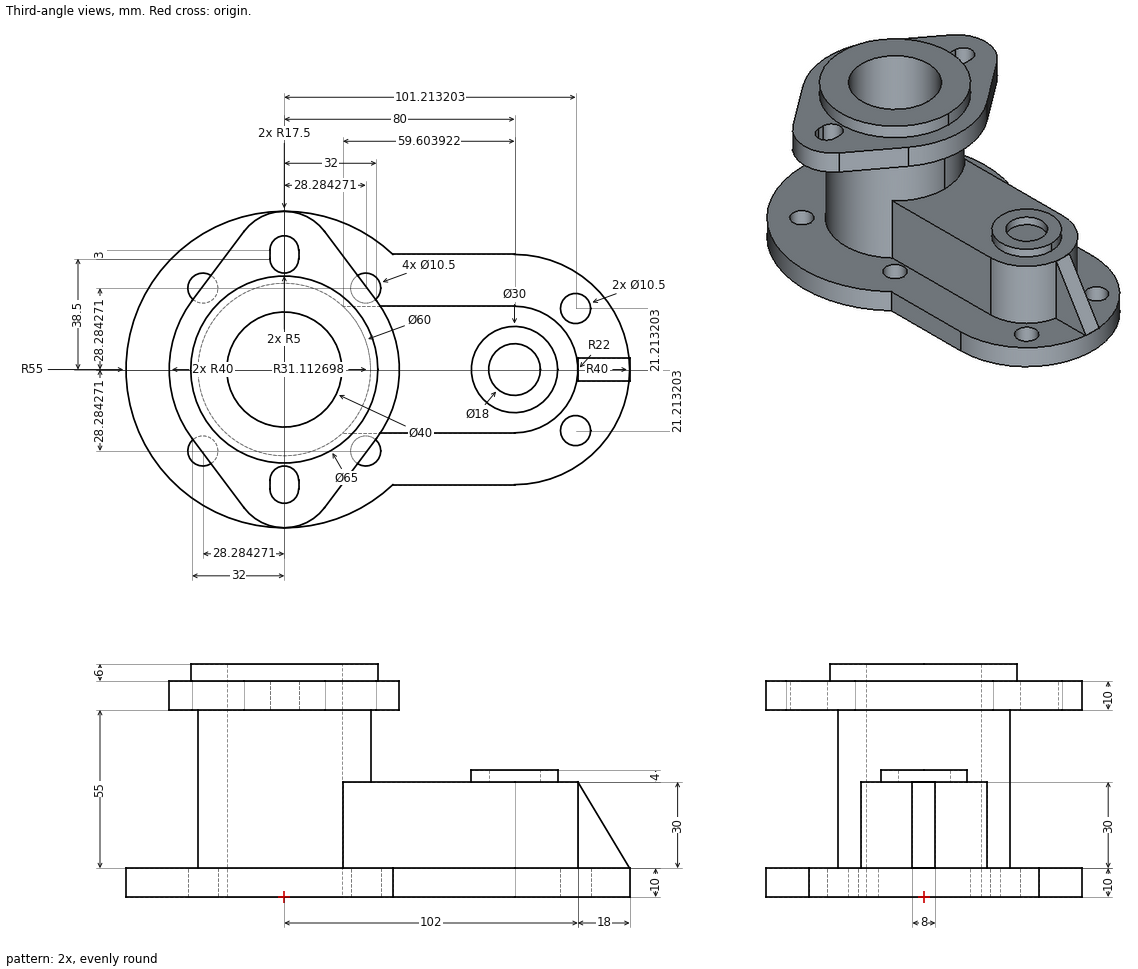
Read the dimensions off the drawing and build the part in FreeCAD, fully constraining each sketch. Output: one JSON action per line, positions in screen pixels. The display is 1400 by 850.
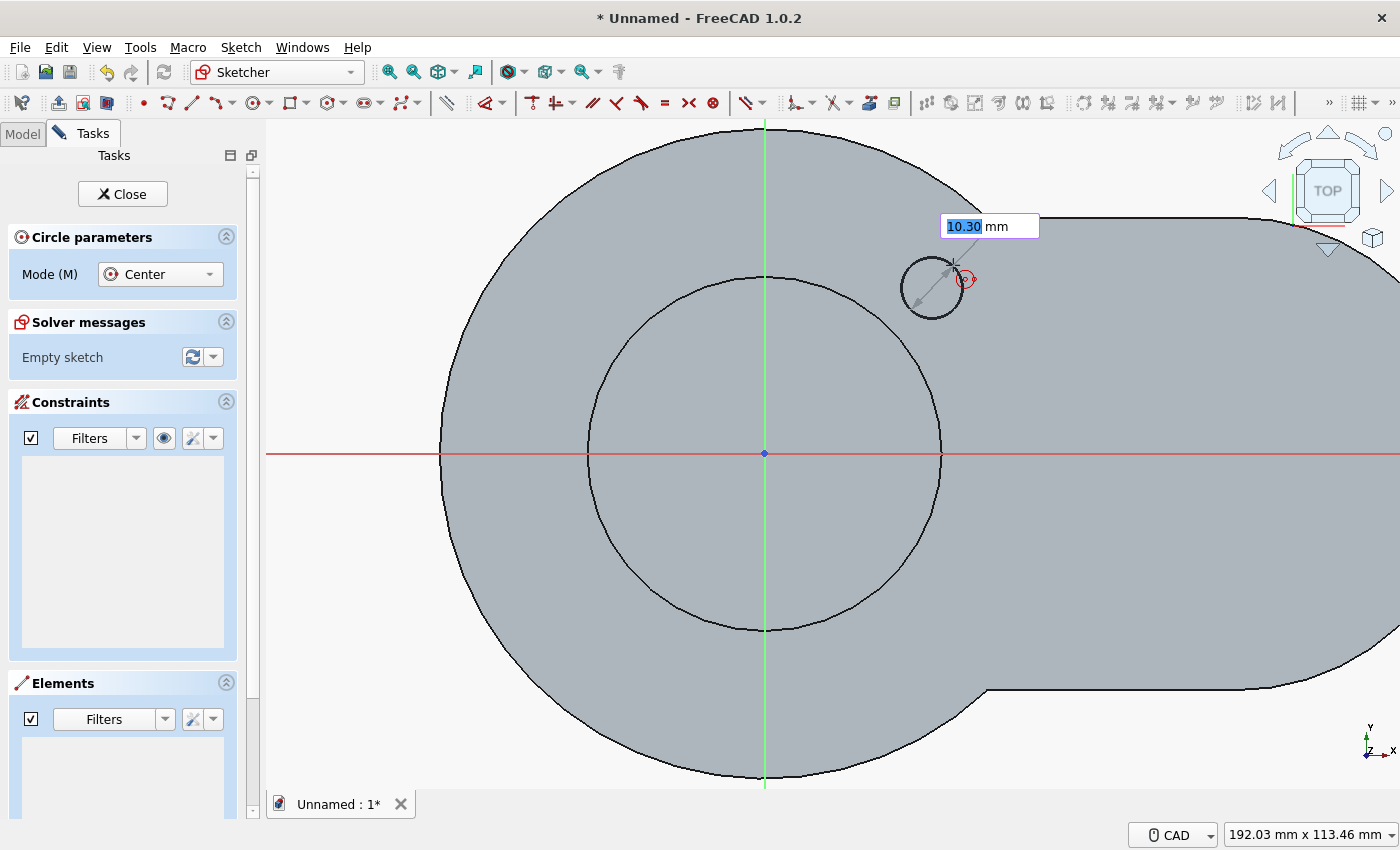
{"action": "type", "text": "10.5"}
{"action": "key", "text": "Return"}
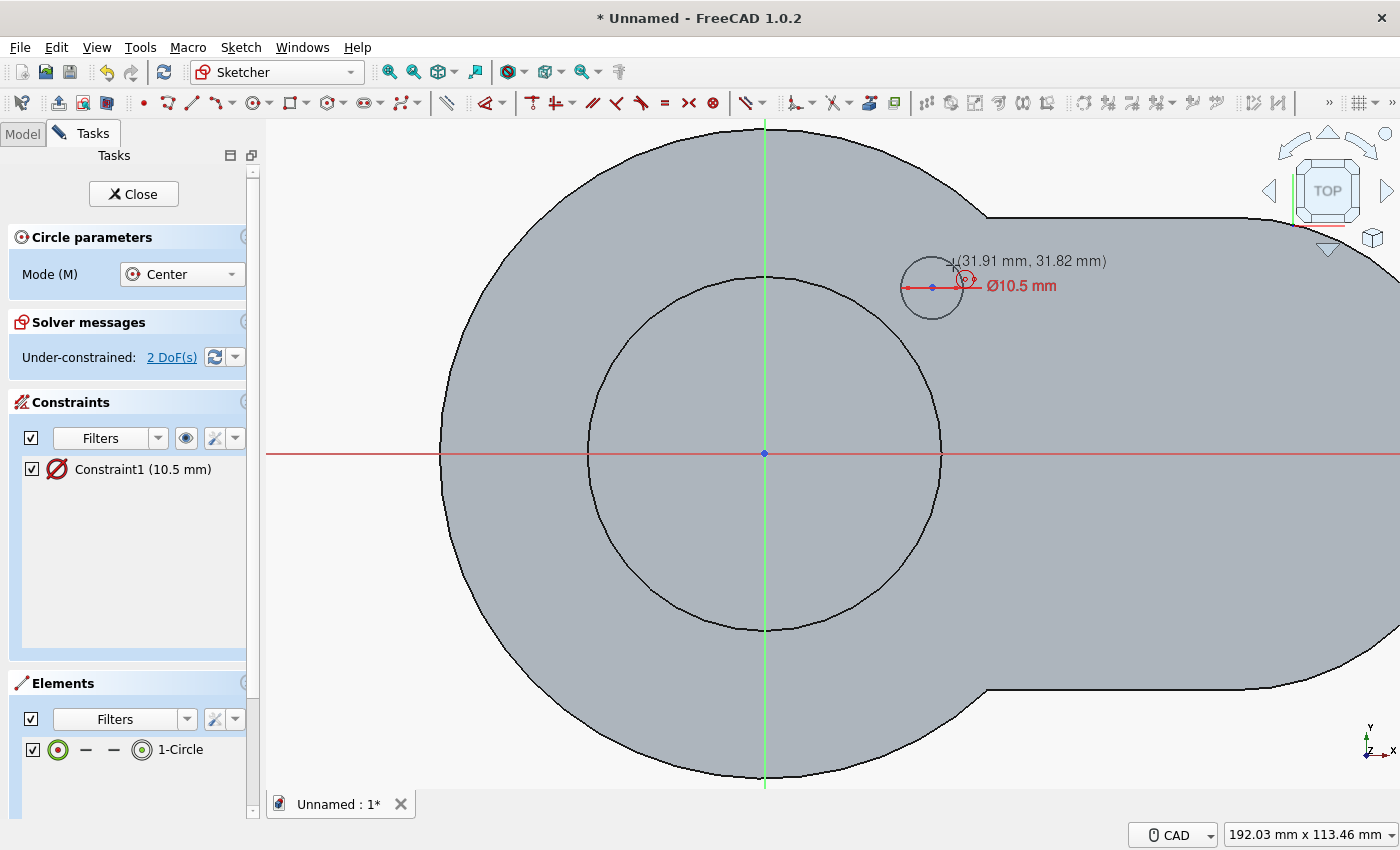
{"action": "left_click", "coordinate": [932, 621]}
{"action": "mouse_move", "coordinate": [953, 599]}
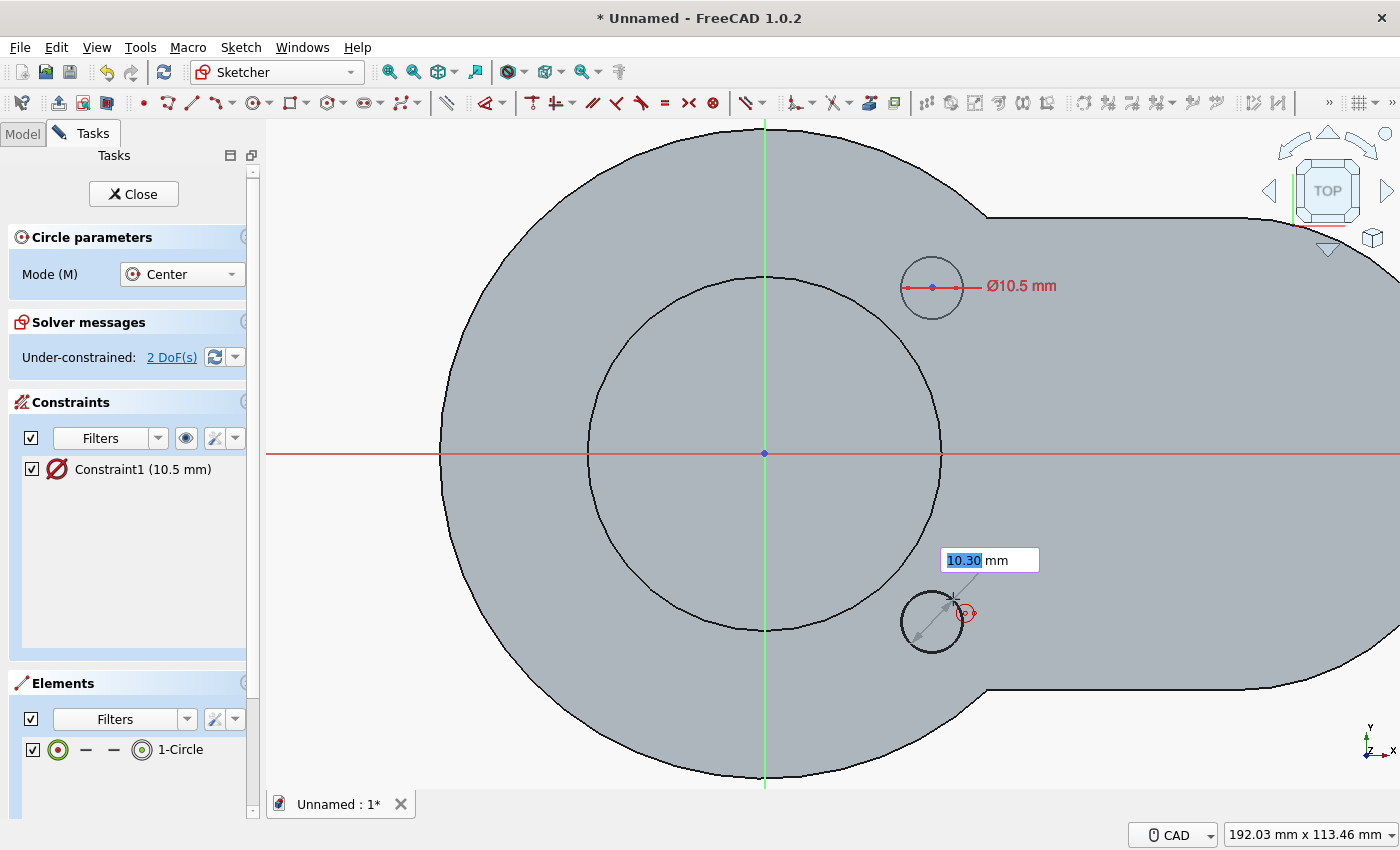
{"action": "type", "text": "10.5"}
{"action": "key", "text": "Return"}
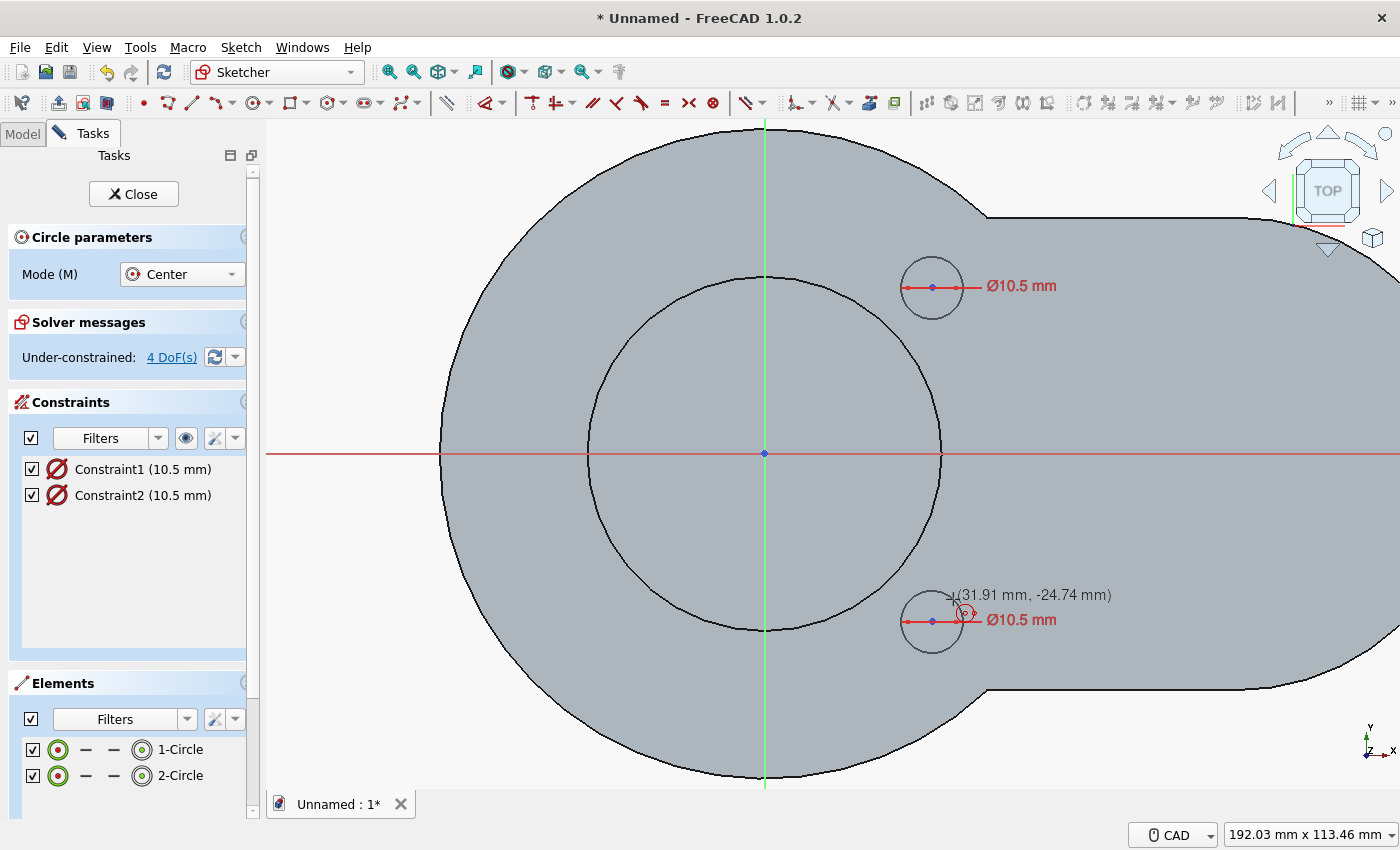
{"action": "left_click", "coordinate": [598, 621]}
{"action": "mouse_move", "coordinate": [619, 599]}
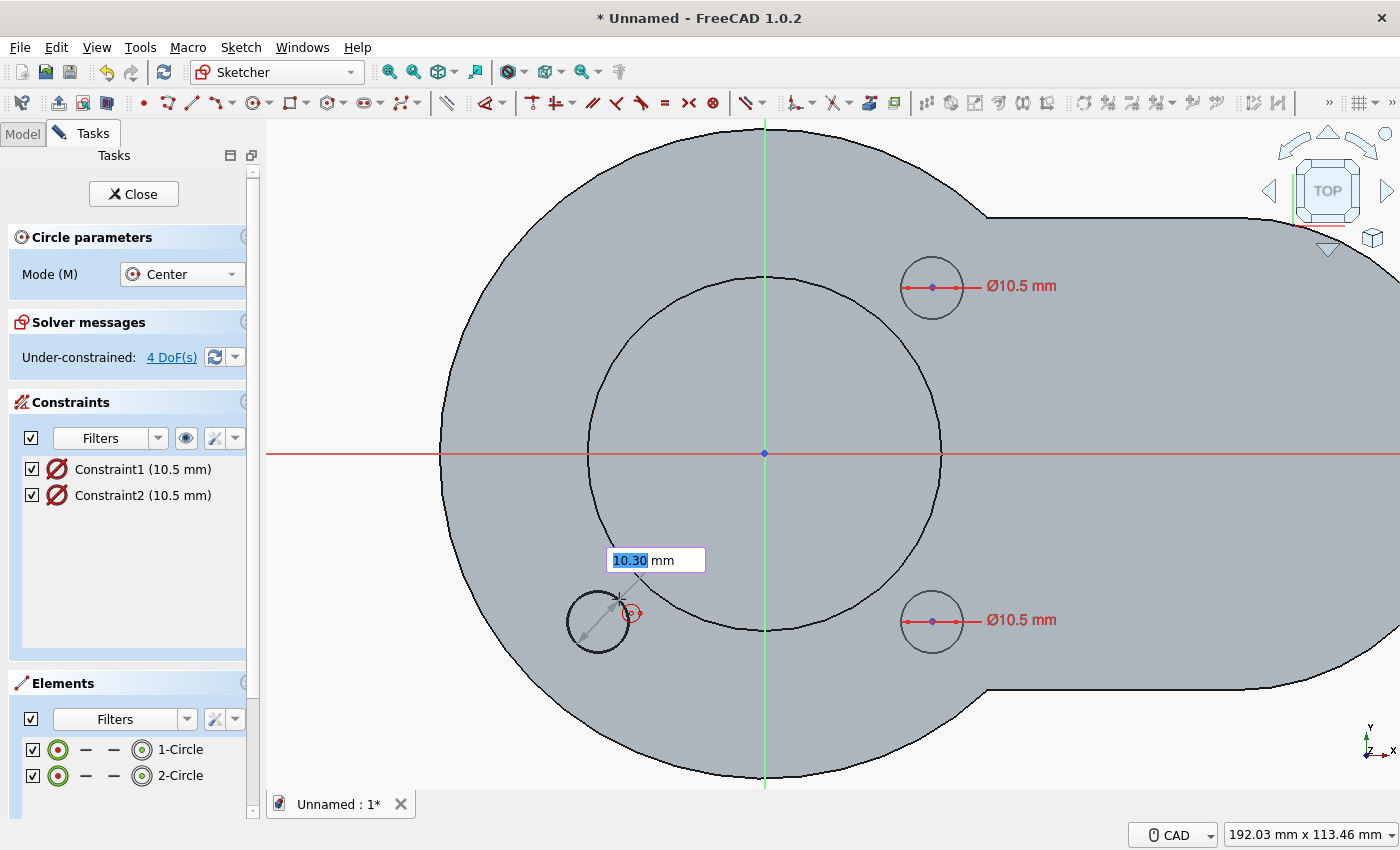
{"action": "type", "text": "10.5"}
{"action": "key", "text": "Return"}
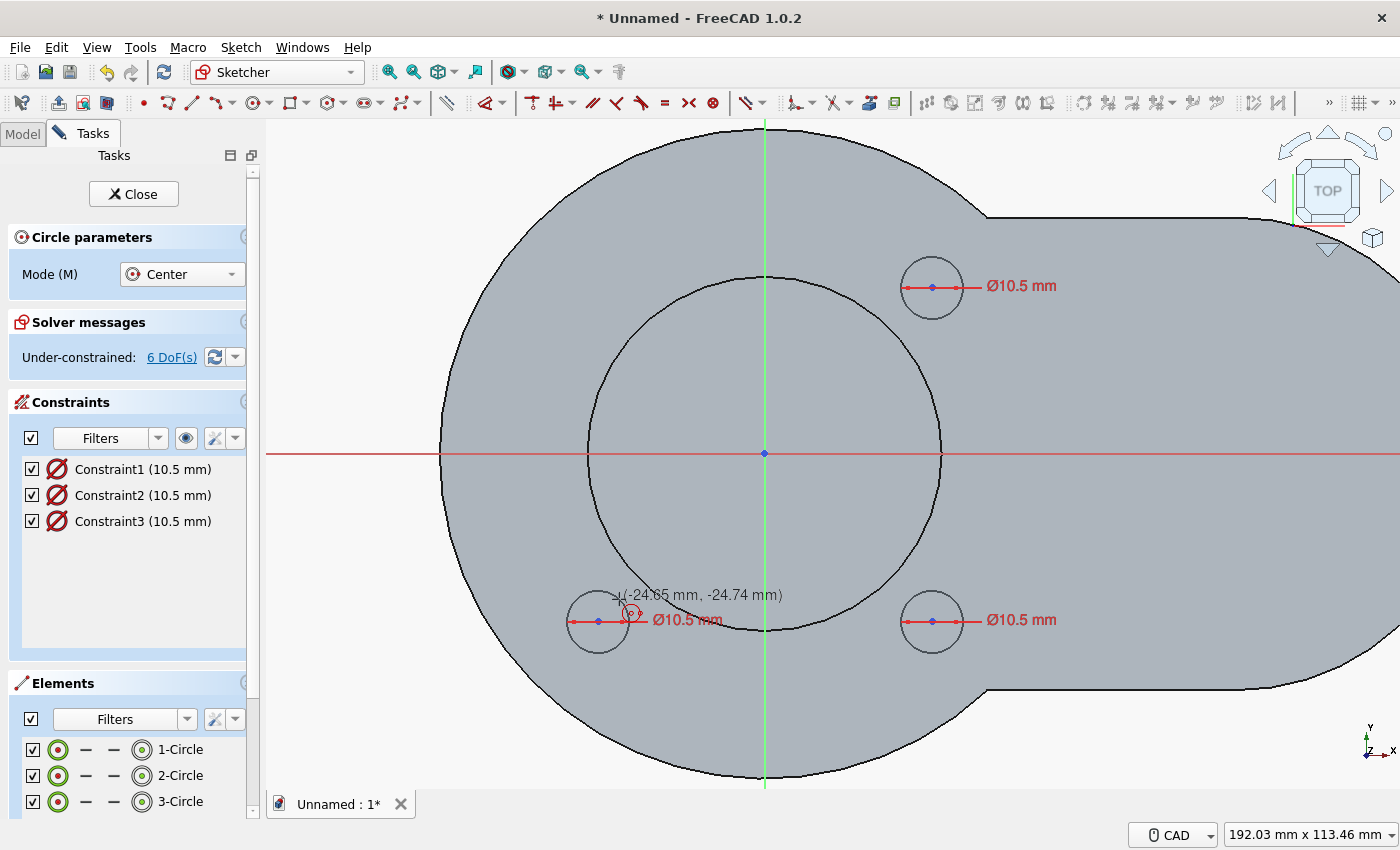
{"action": "left_click", "coordinate": [598, 287]}
{"action": "mouse_move", "coordinate": [619, 265]}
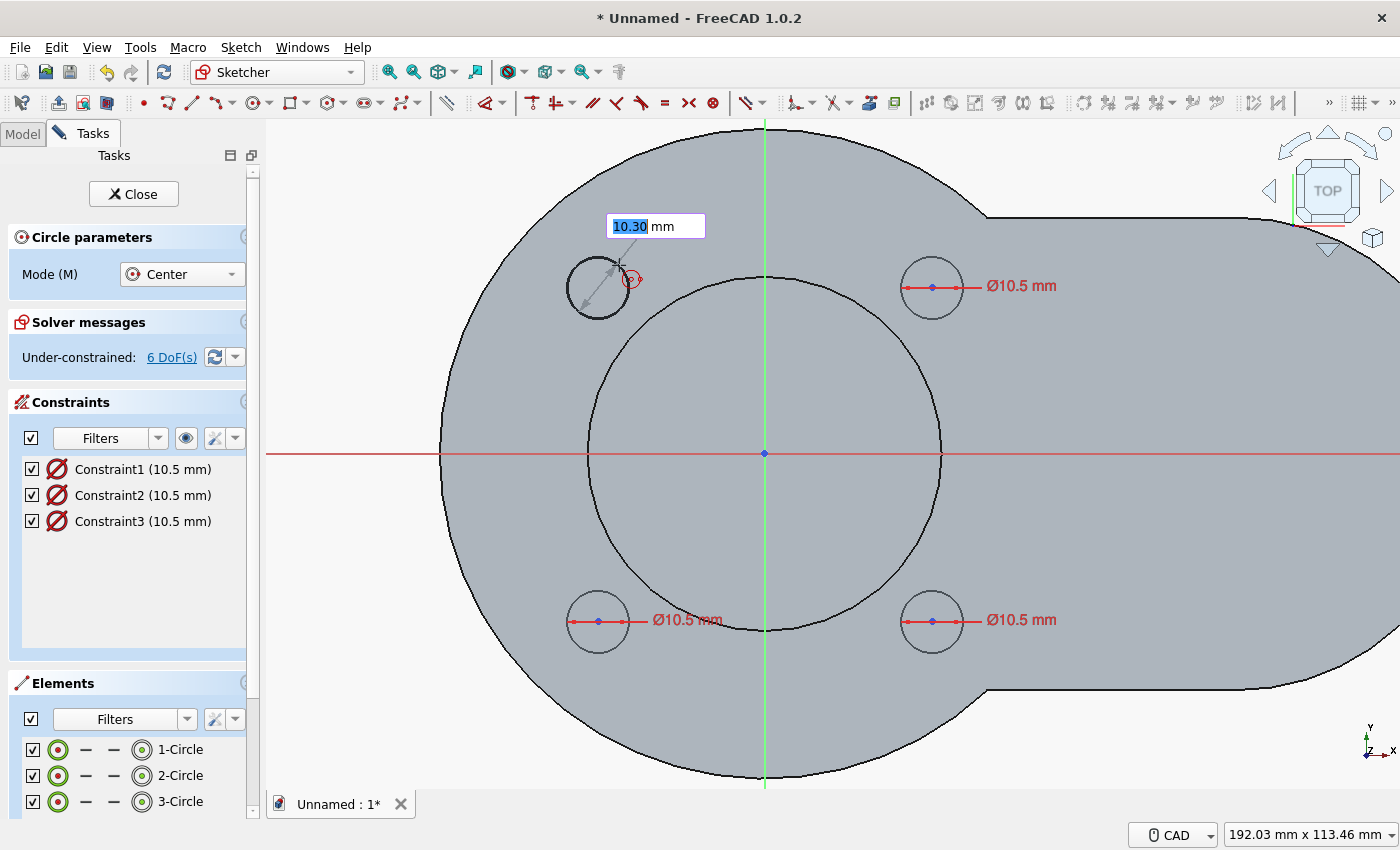
{"action": "type", "text": "10.5"}
{"action": "key", "text": "Return"}
{"action": "key", "text": "Escape"}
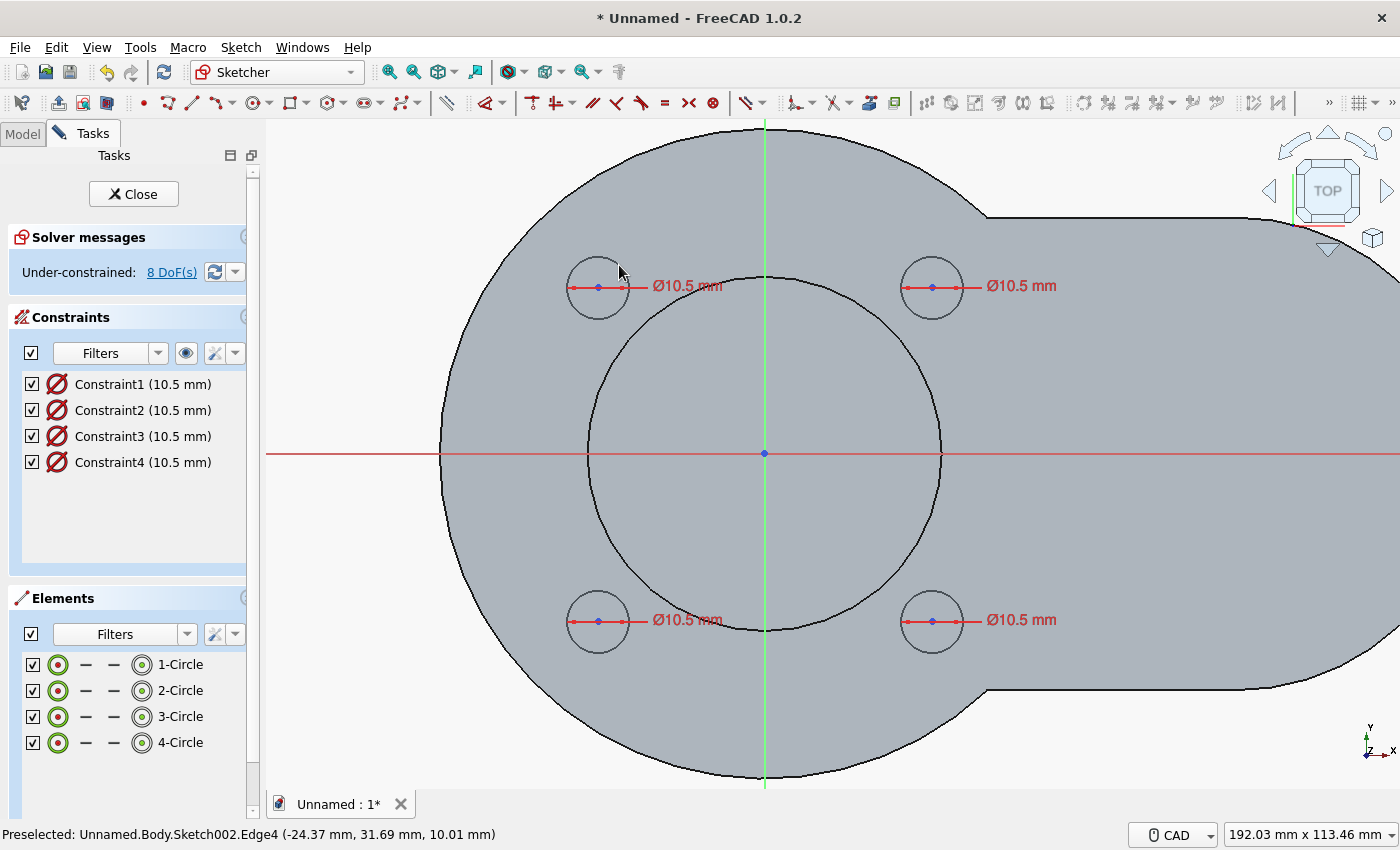
{"action": "left_click", "coordinate": [932, 288]}